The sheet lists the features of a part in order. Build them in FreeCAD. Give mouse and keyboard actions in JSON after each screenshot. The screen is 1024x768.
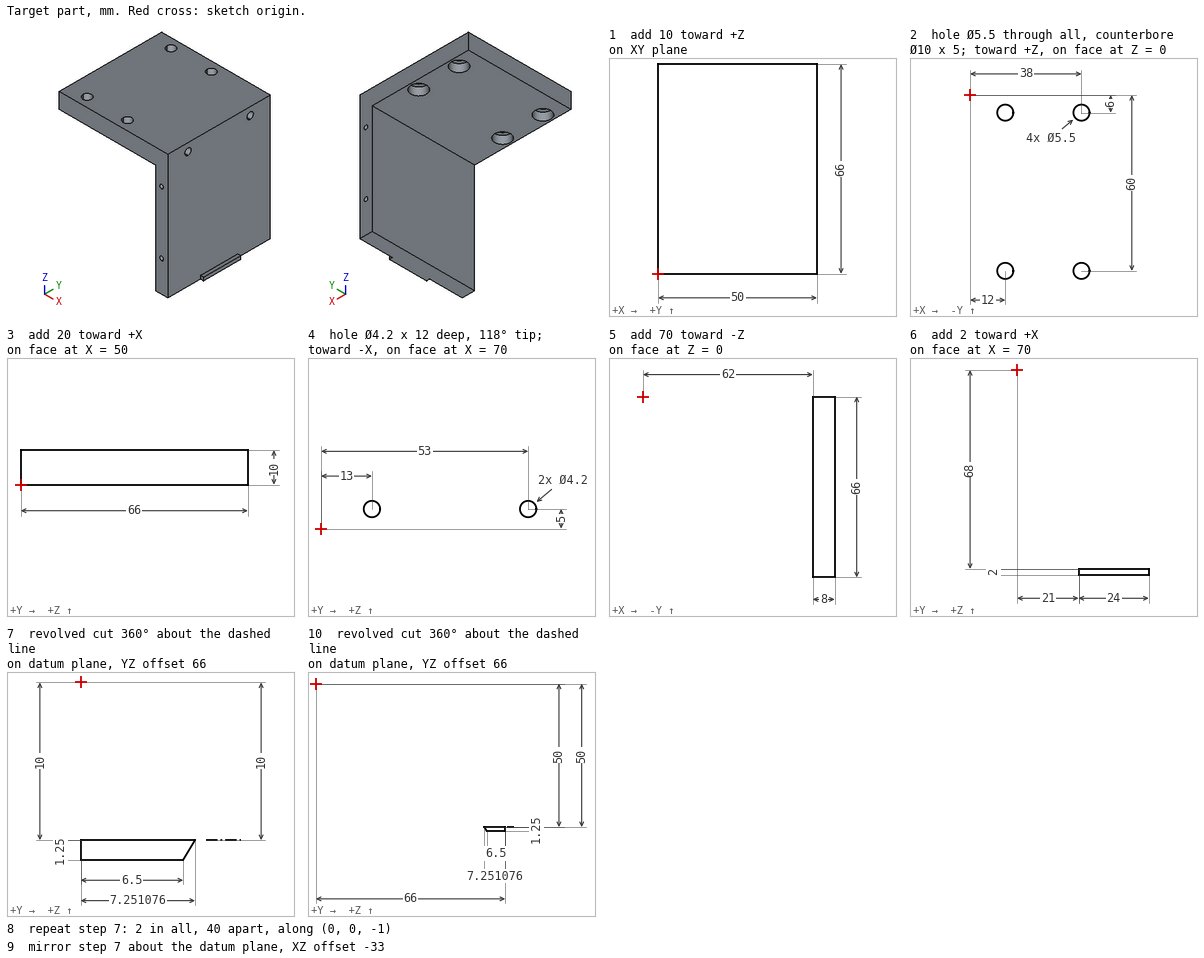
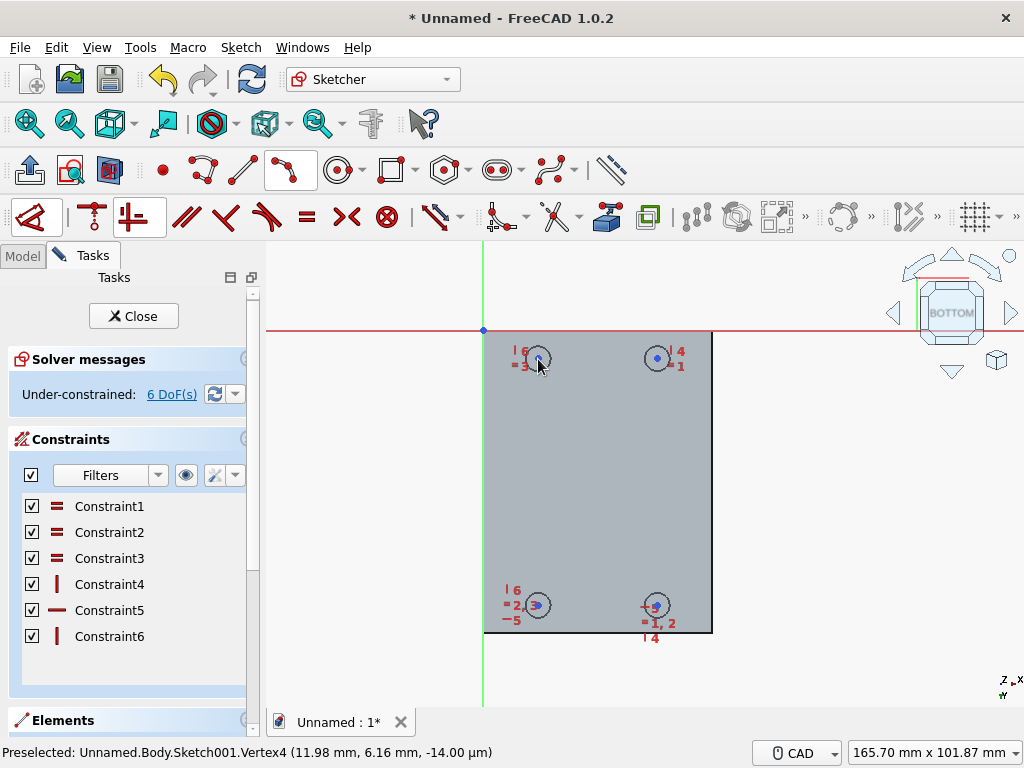
{"action": "left_click", "coordinate": [657, 359]}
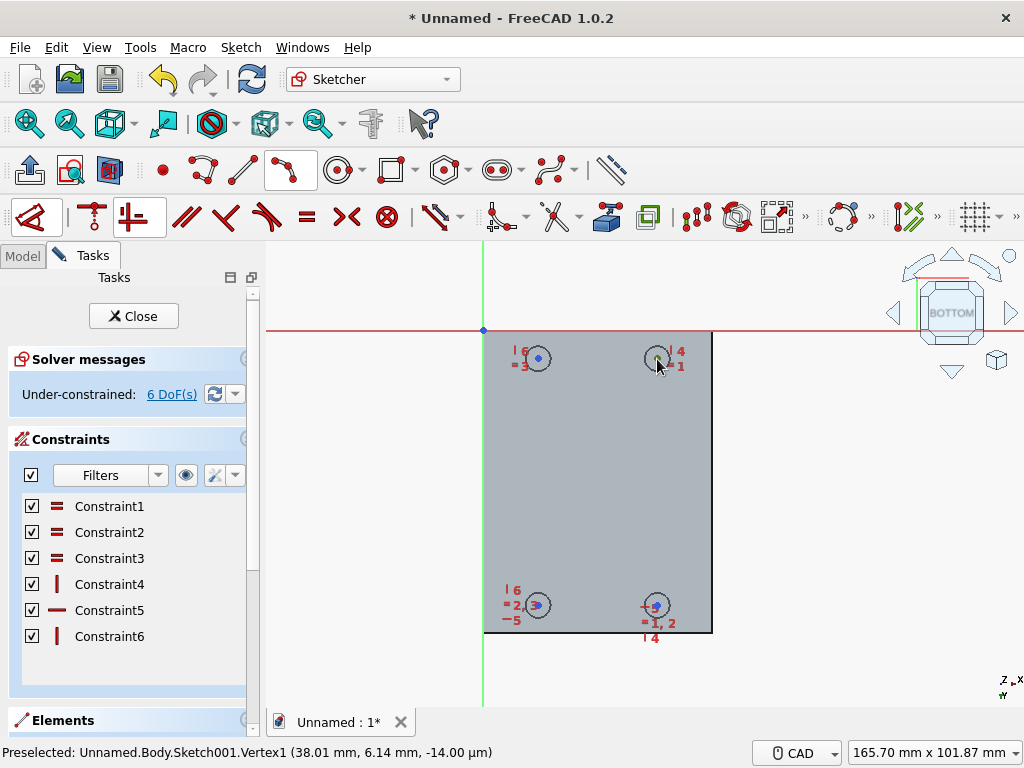
{"action": "left_click", "coordinate": [538, 359]}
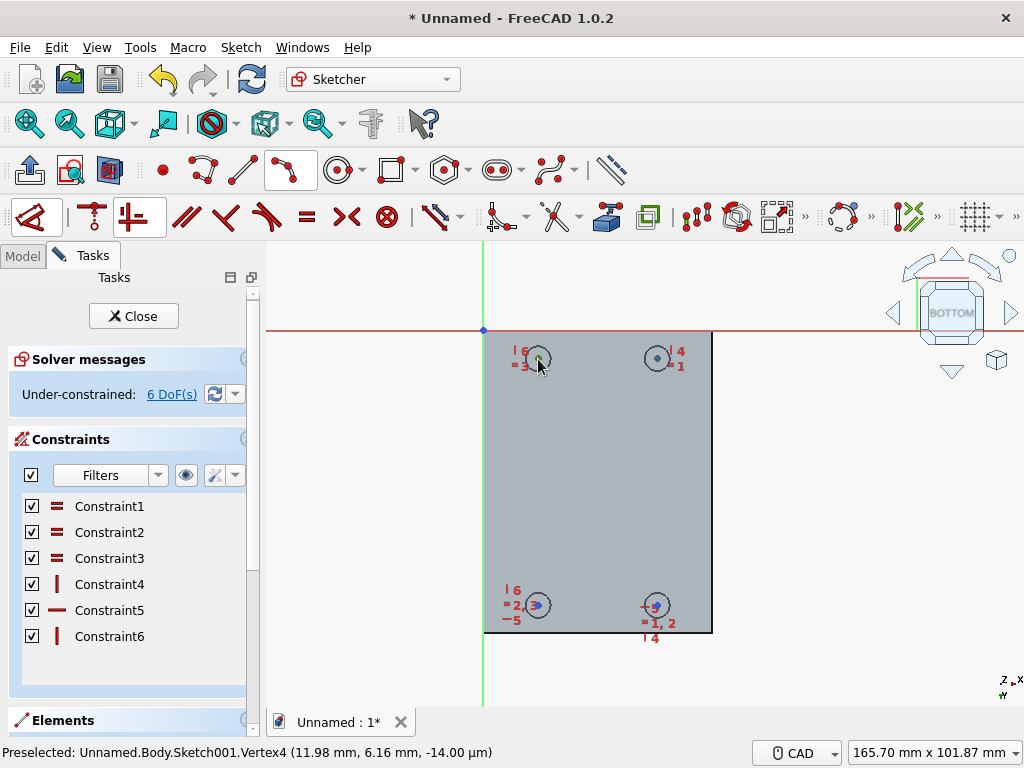
{"action": "key", "text": "h"}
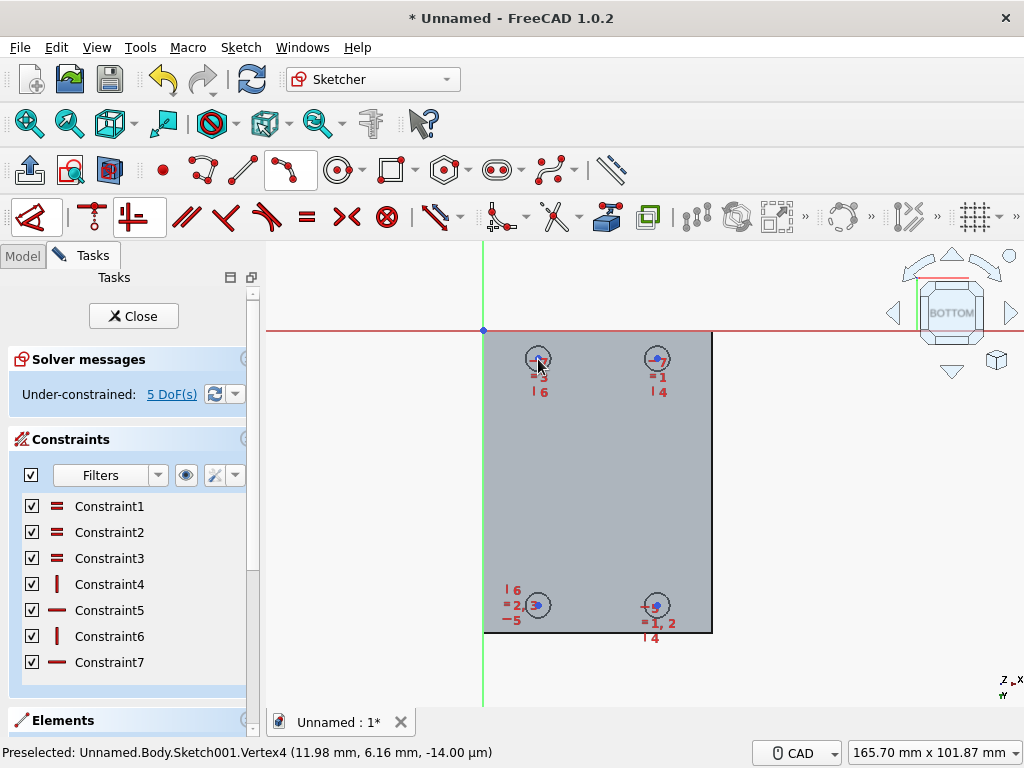
{"action": "scroll", "coordinate": [666, 350], "scroll_direction": "up", "scroll_amount": 3}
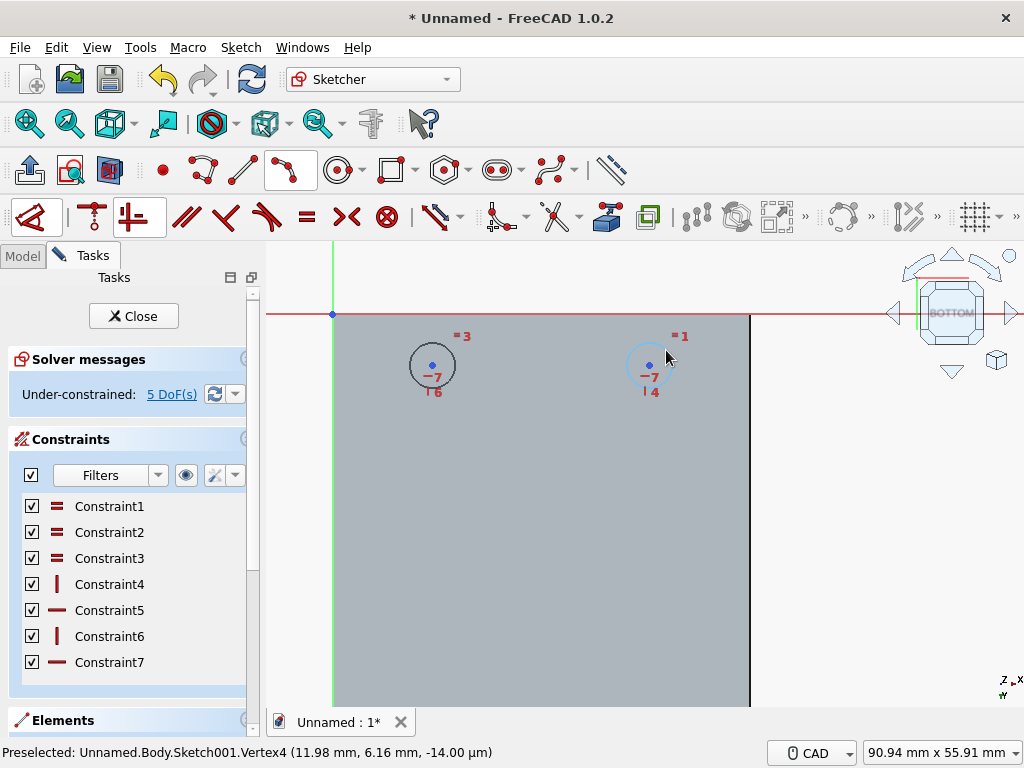
{"action": "left_click", "coordinate": [666, 350]}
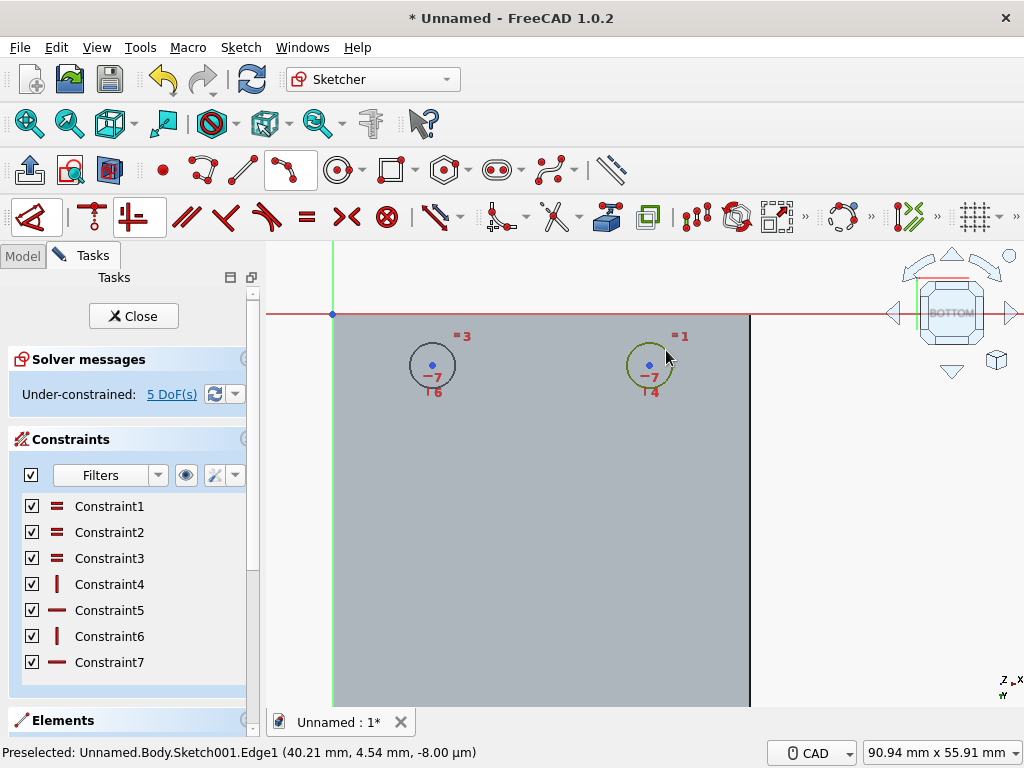
{"action": "key", "text": "k o"}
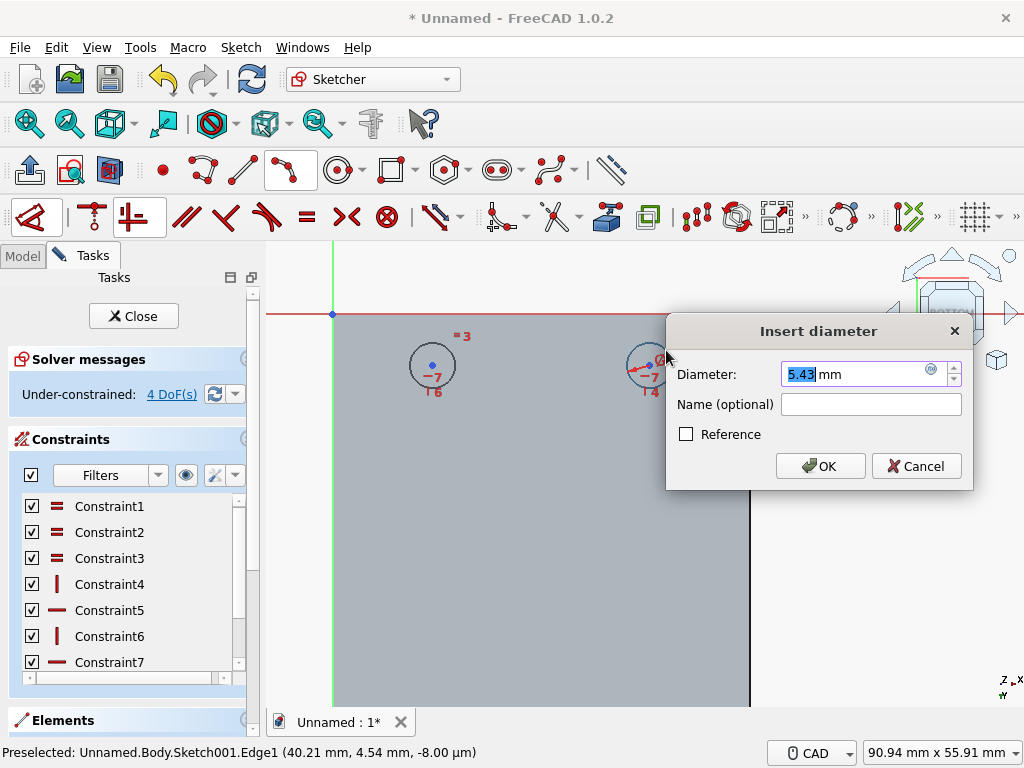
{"action": "type", "text": "5.5"}
{"action": "key", "text": "Return"}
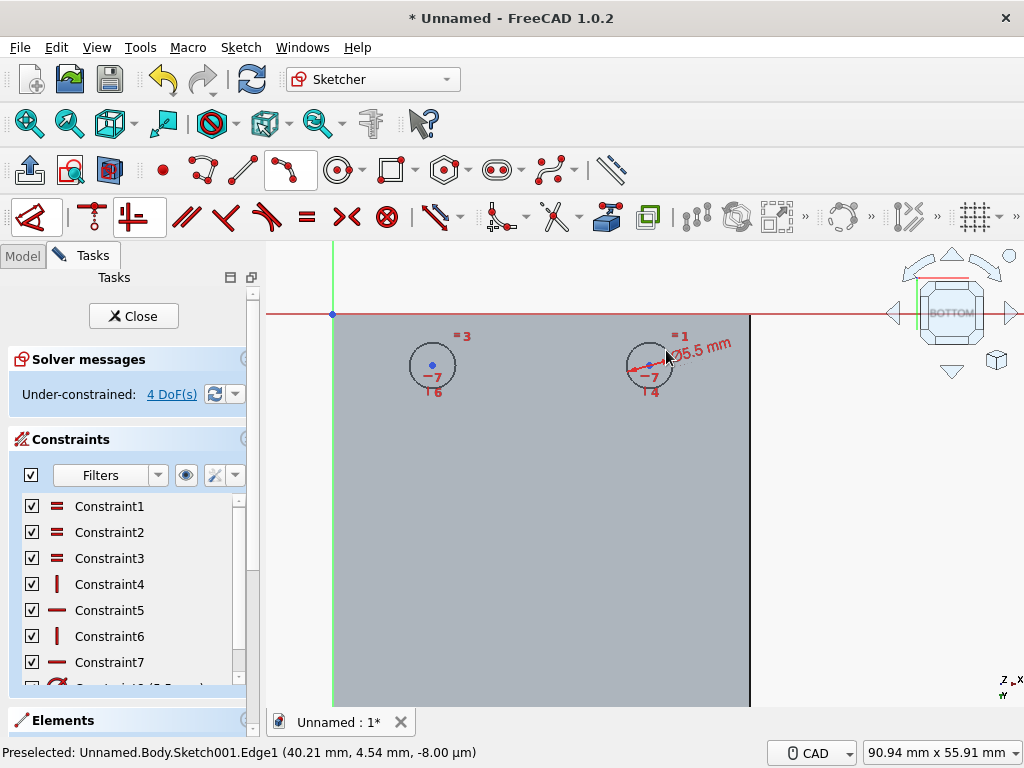
{"action": "left_click", "coordinate": [650, 366]}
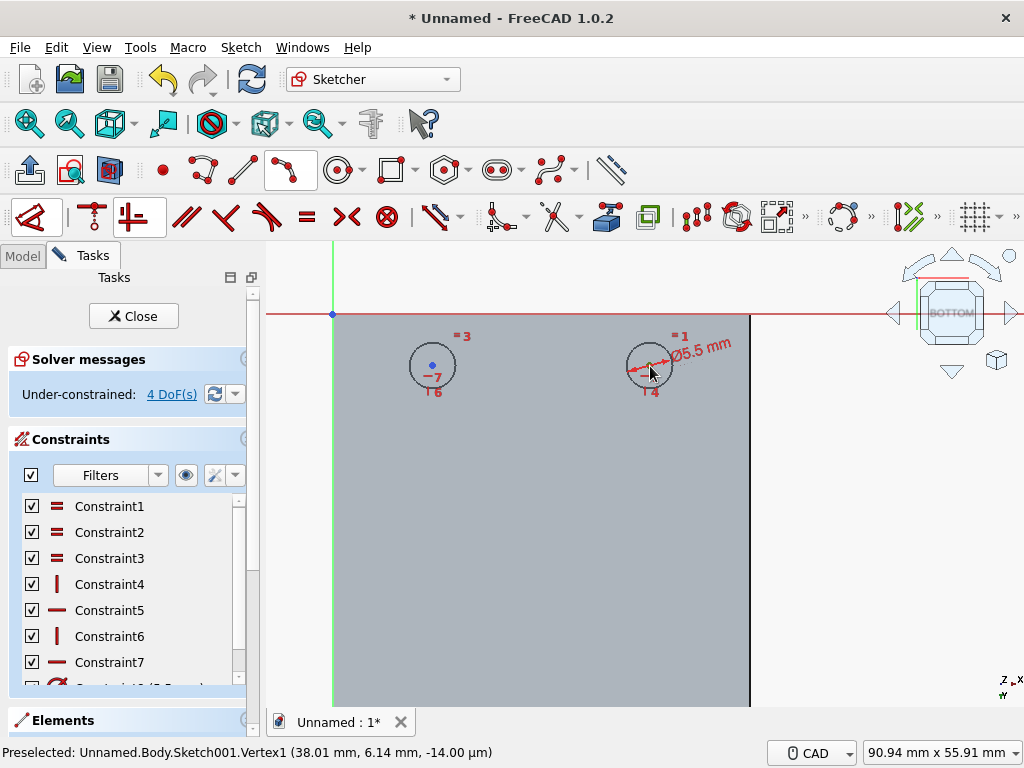
{"action": "key", "text": "i"}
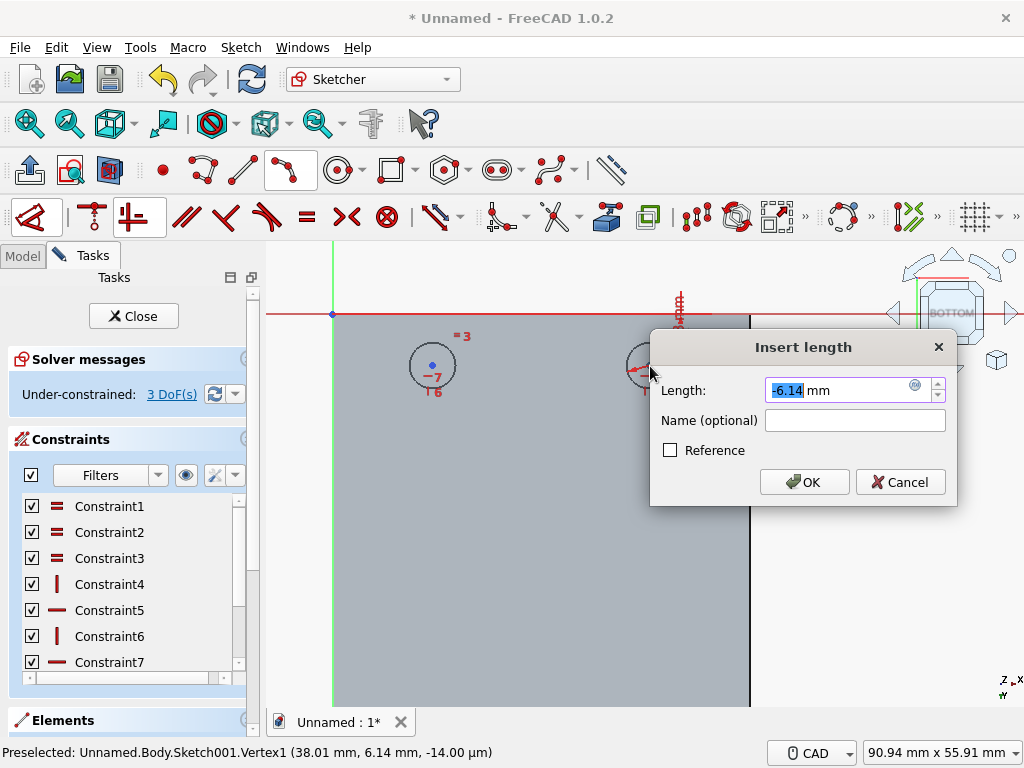
{"action": "type", "text": "-6"}
{"action": "key", "text": "Return"}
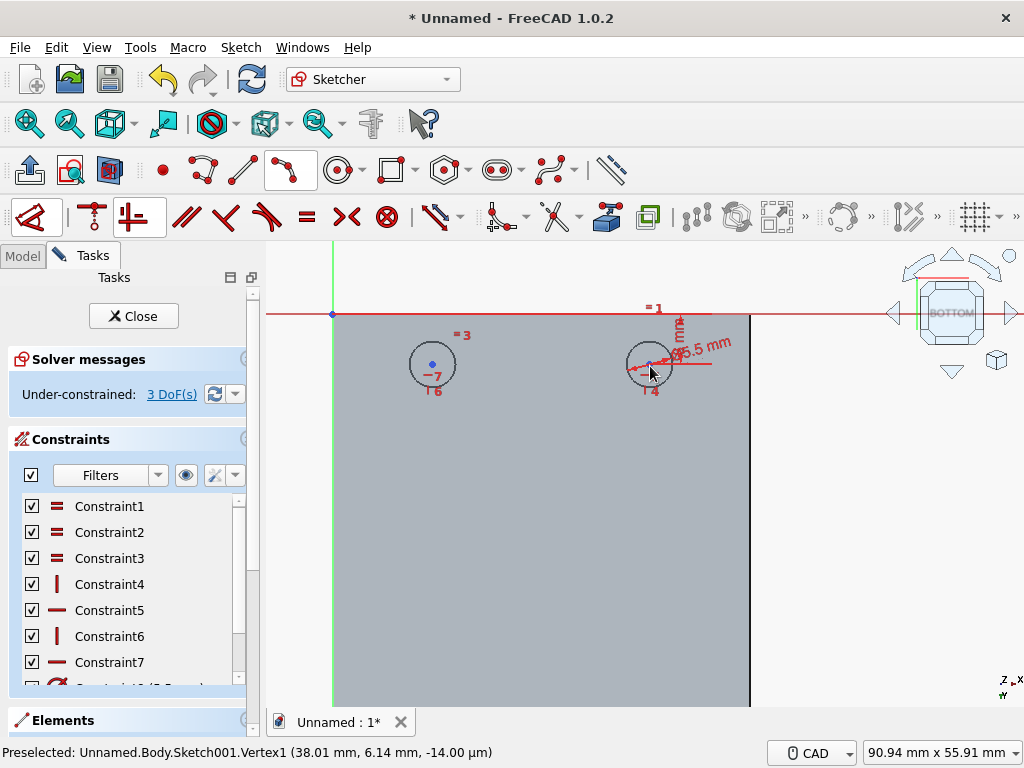
{"action": "left_click", "coordinate": [650, 364]}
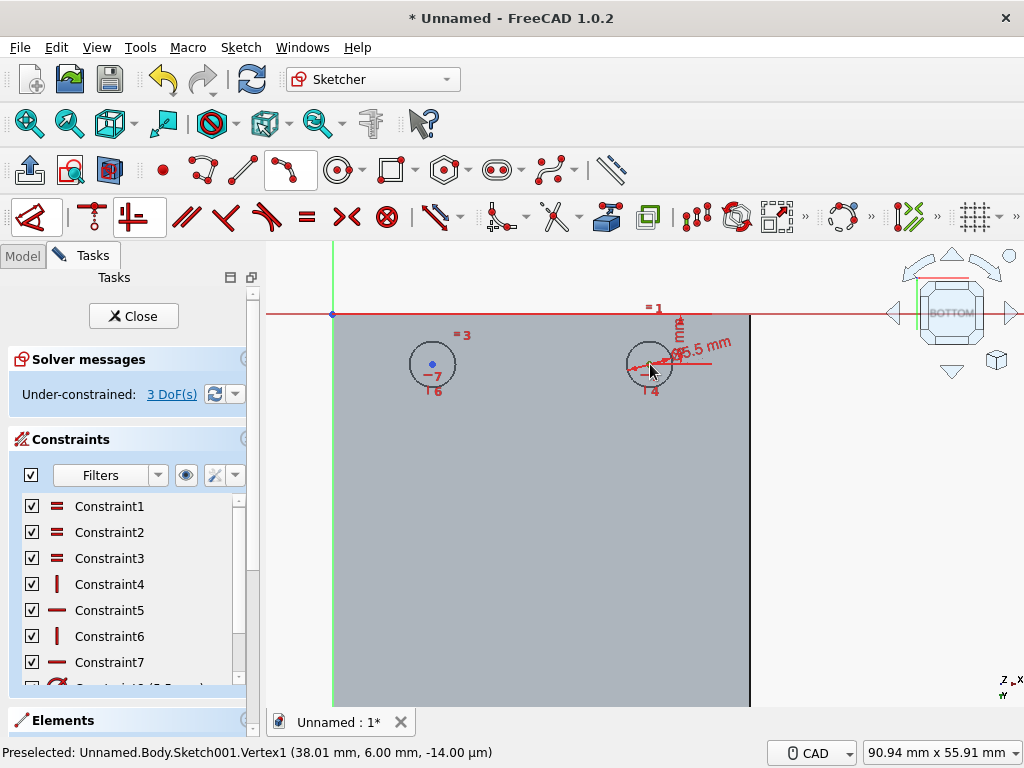
{"action": "key", "text": "l"}